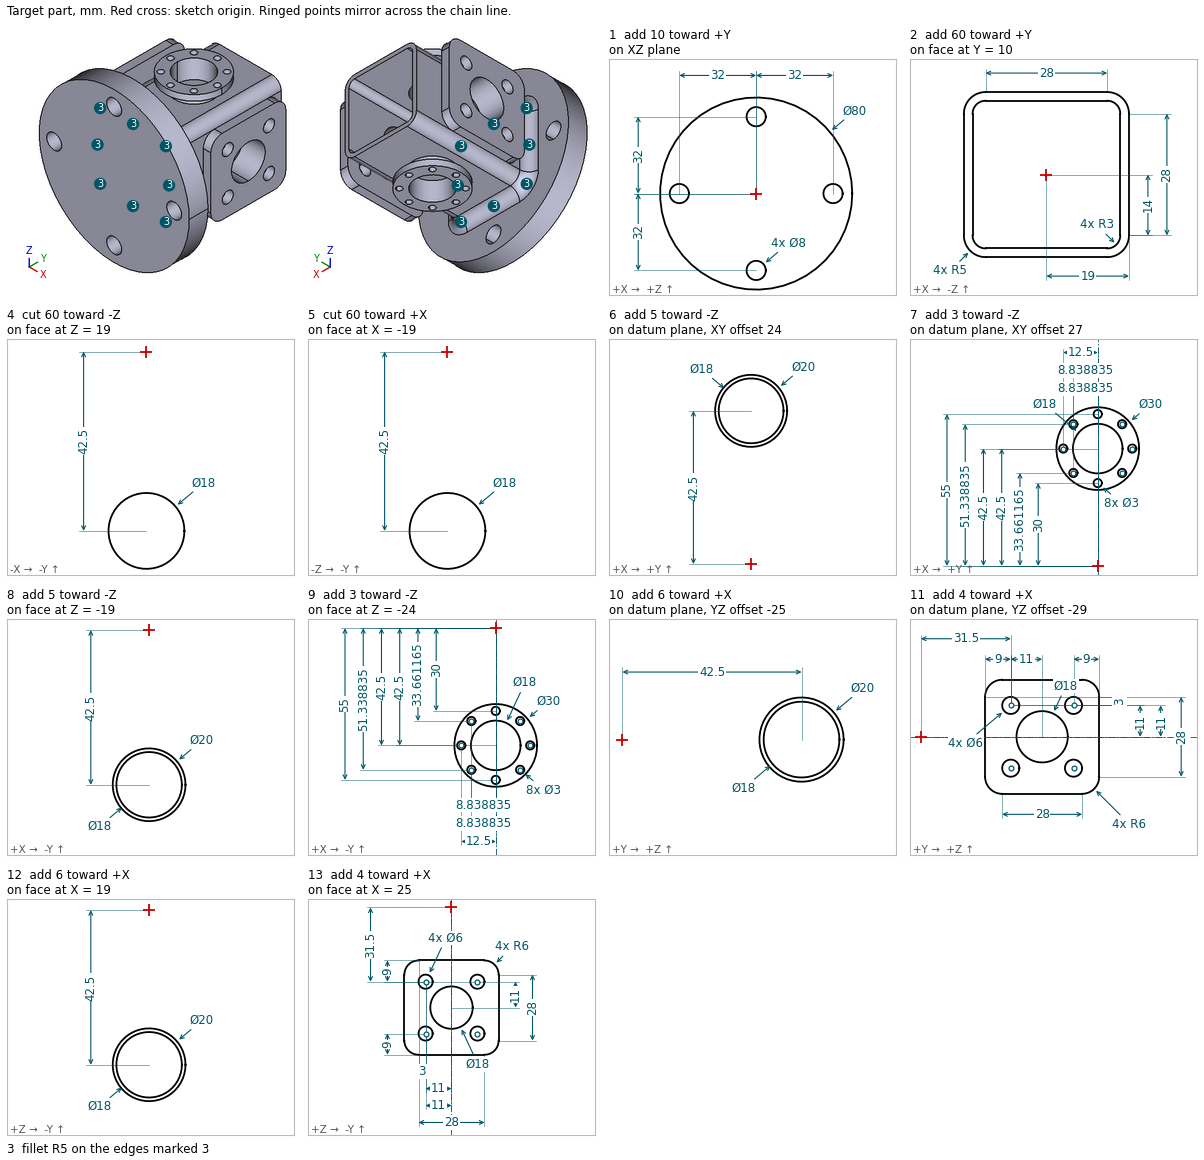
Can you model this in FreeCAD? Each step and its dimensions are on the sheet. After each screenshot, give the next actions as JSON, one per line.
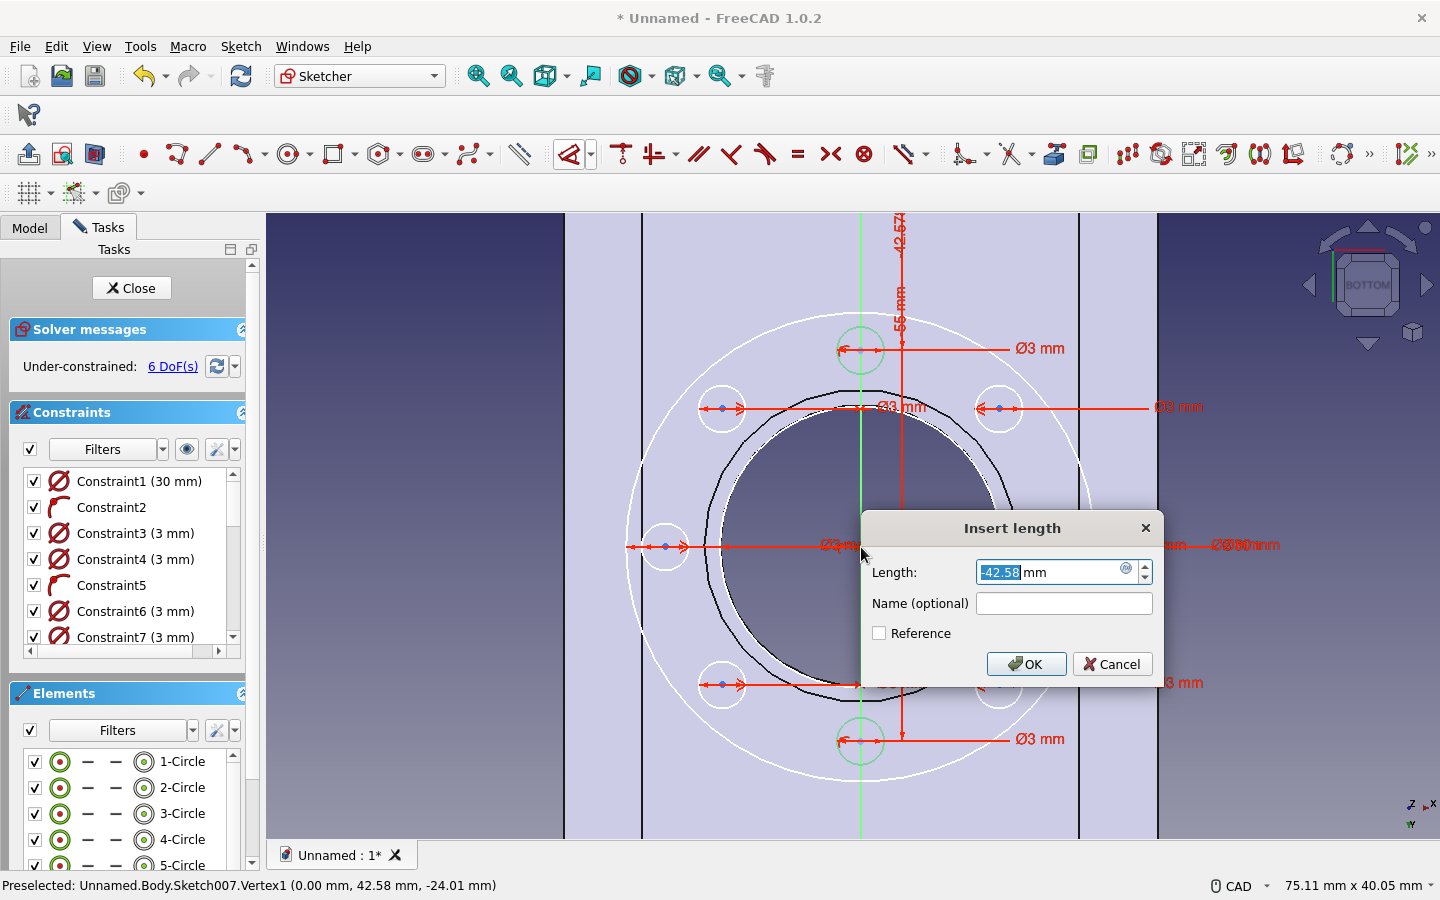
{"action": "type", "text": "-42.5"}
{"action": "key", "text": "Return"}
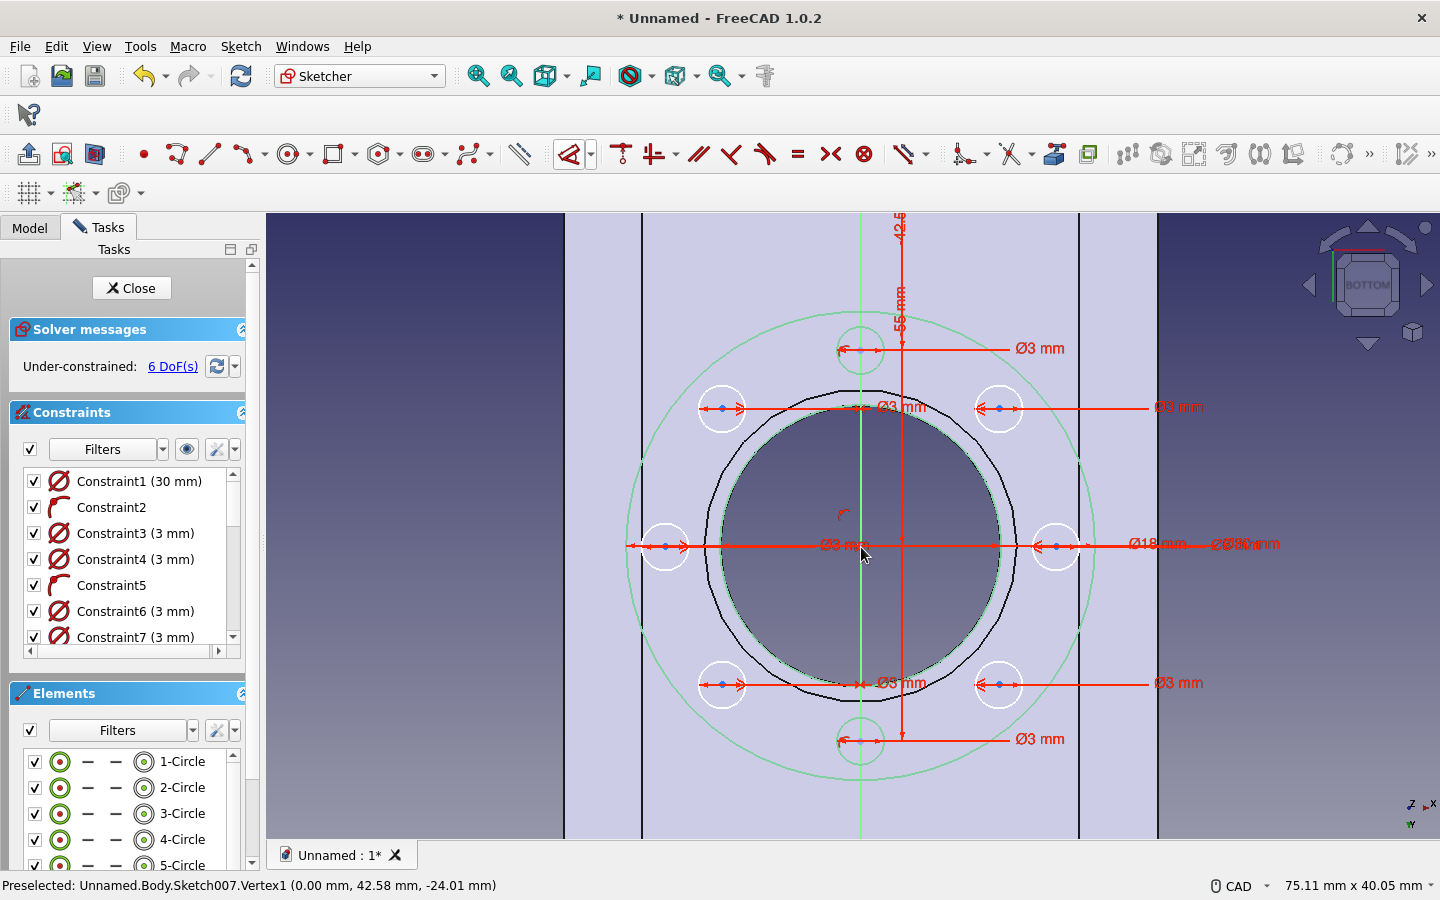
{"action": "left_click", "coordinate": [665, 547]}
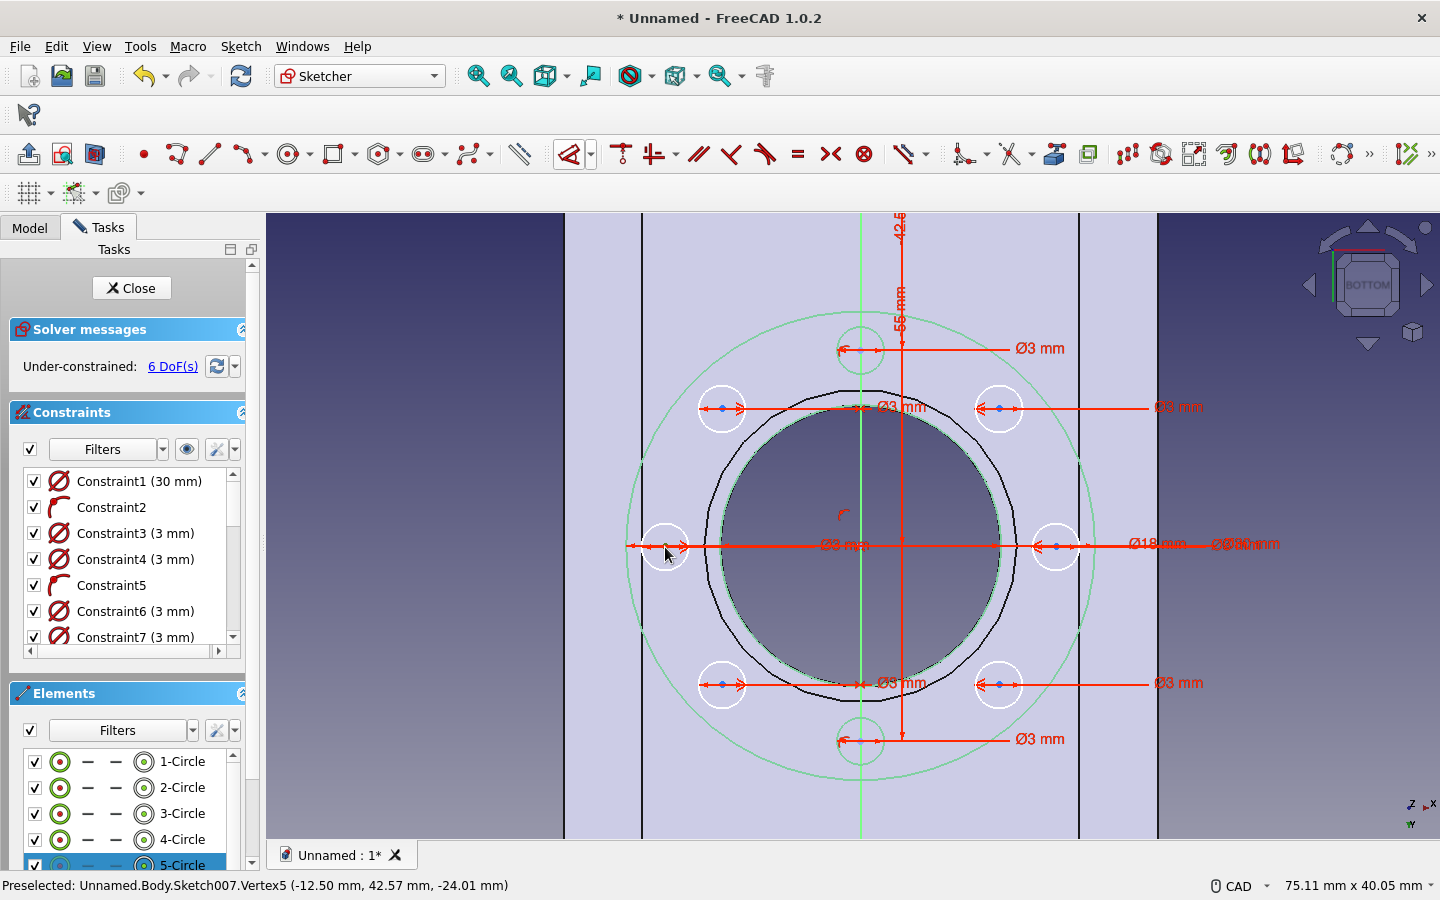
{"action": "key", "text": "l"}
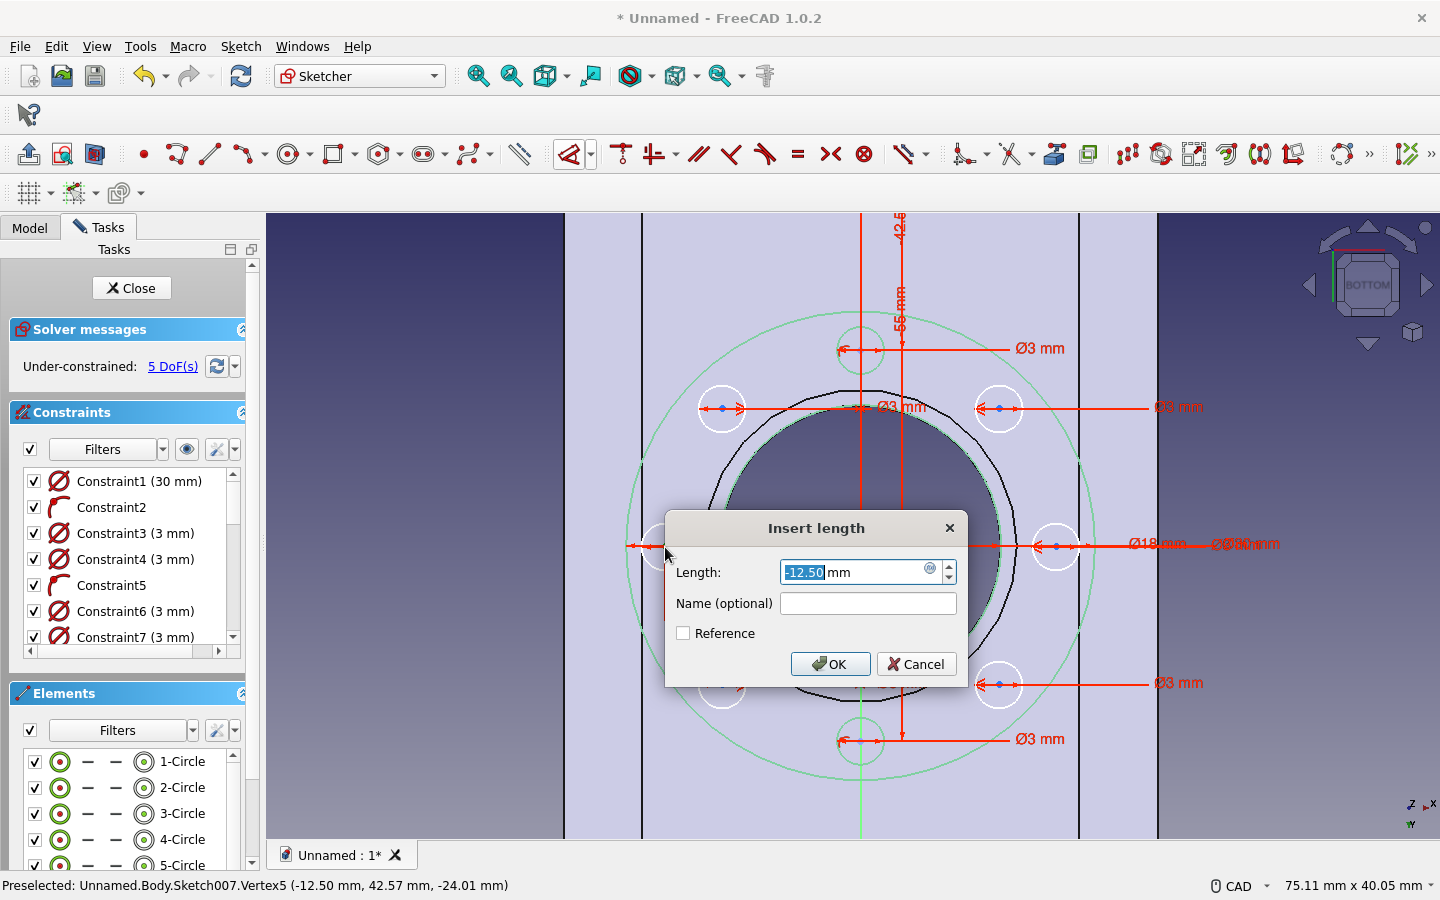
{"action": "type", "text": "-12.5"}
{"action": "key", "text": "Return"}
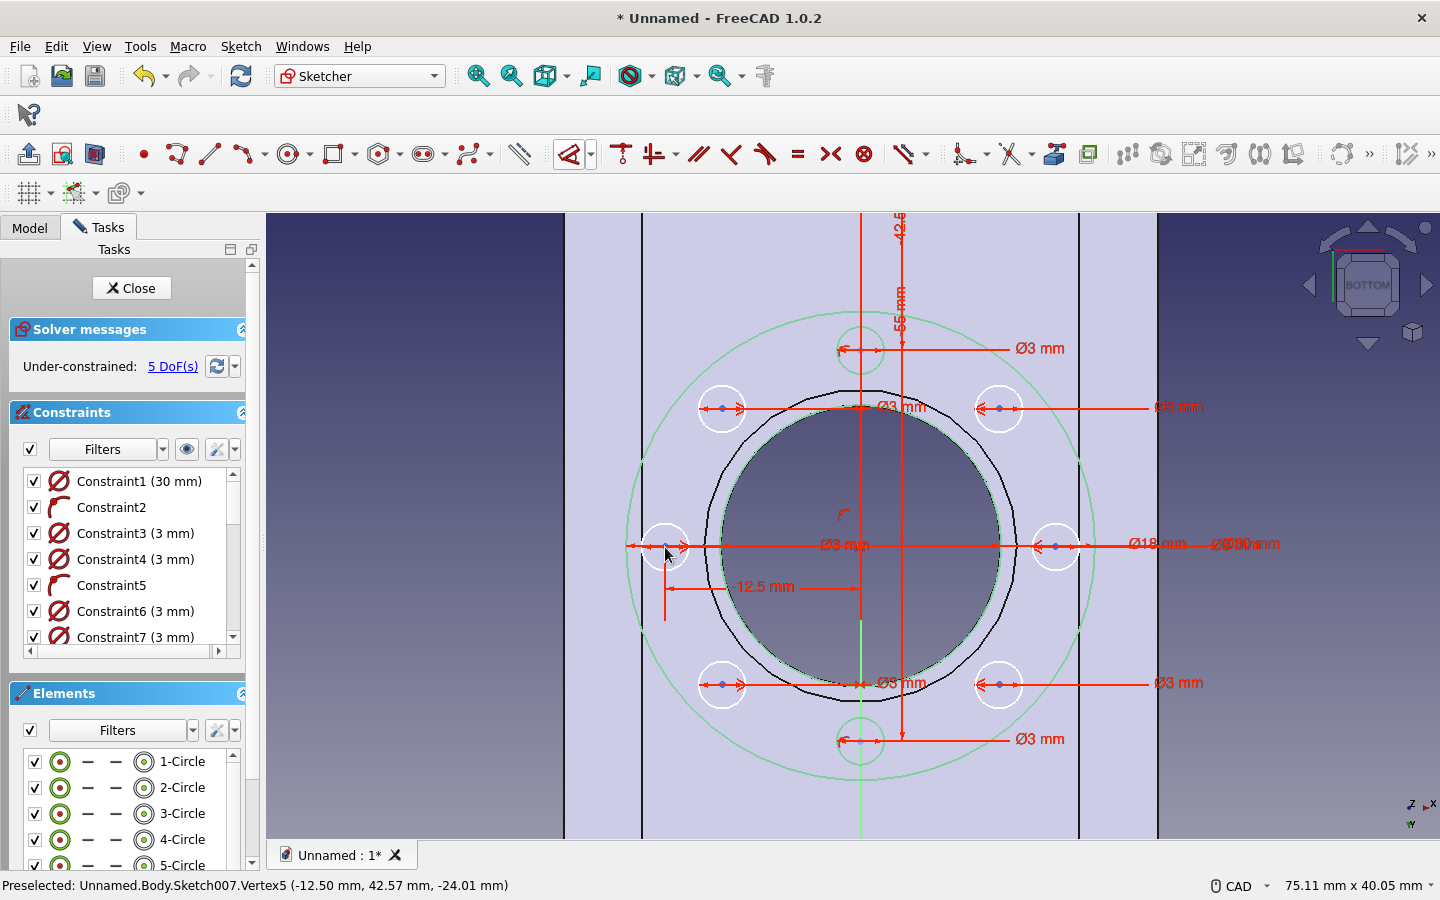
{"action": "left_click", "coordinate": [665, 547]}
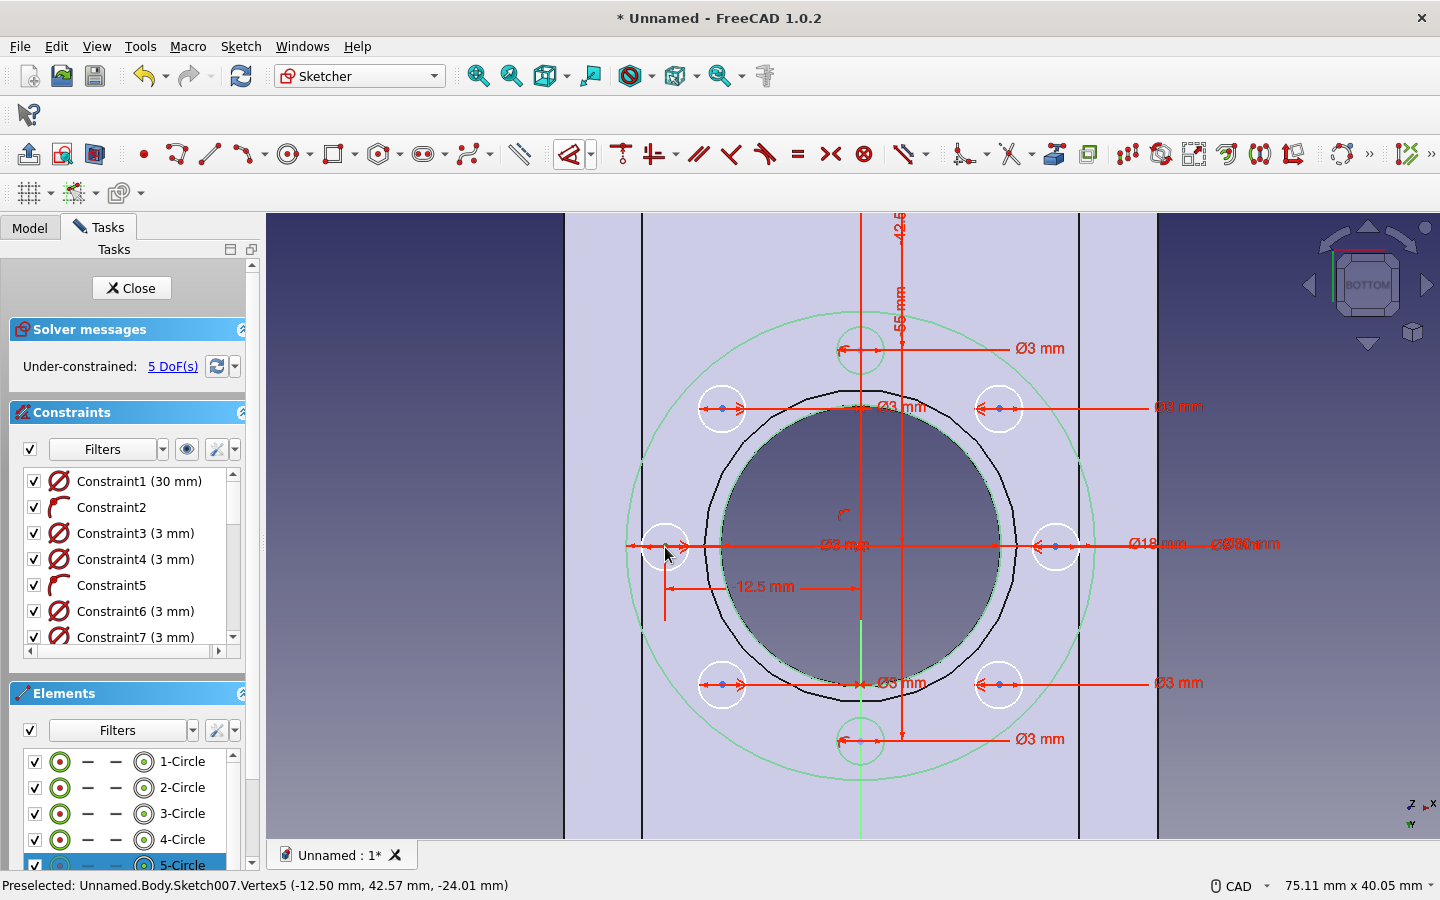
{"action": "key", "text": "i"}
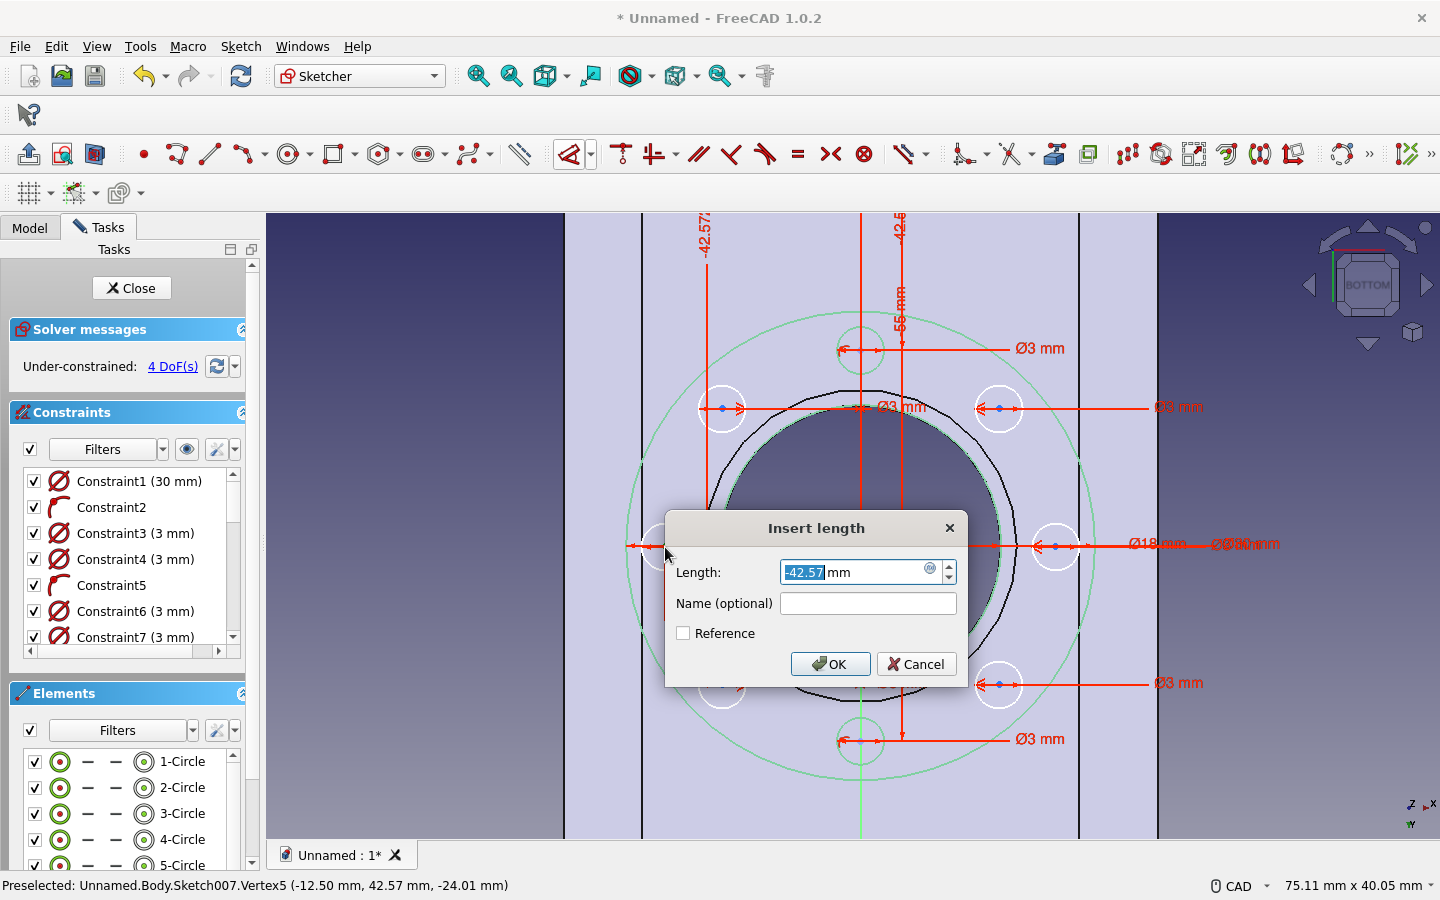
{"action": "type", "text": "-42.5"}
{"action": "key", "text": "Return"}